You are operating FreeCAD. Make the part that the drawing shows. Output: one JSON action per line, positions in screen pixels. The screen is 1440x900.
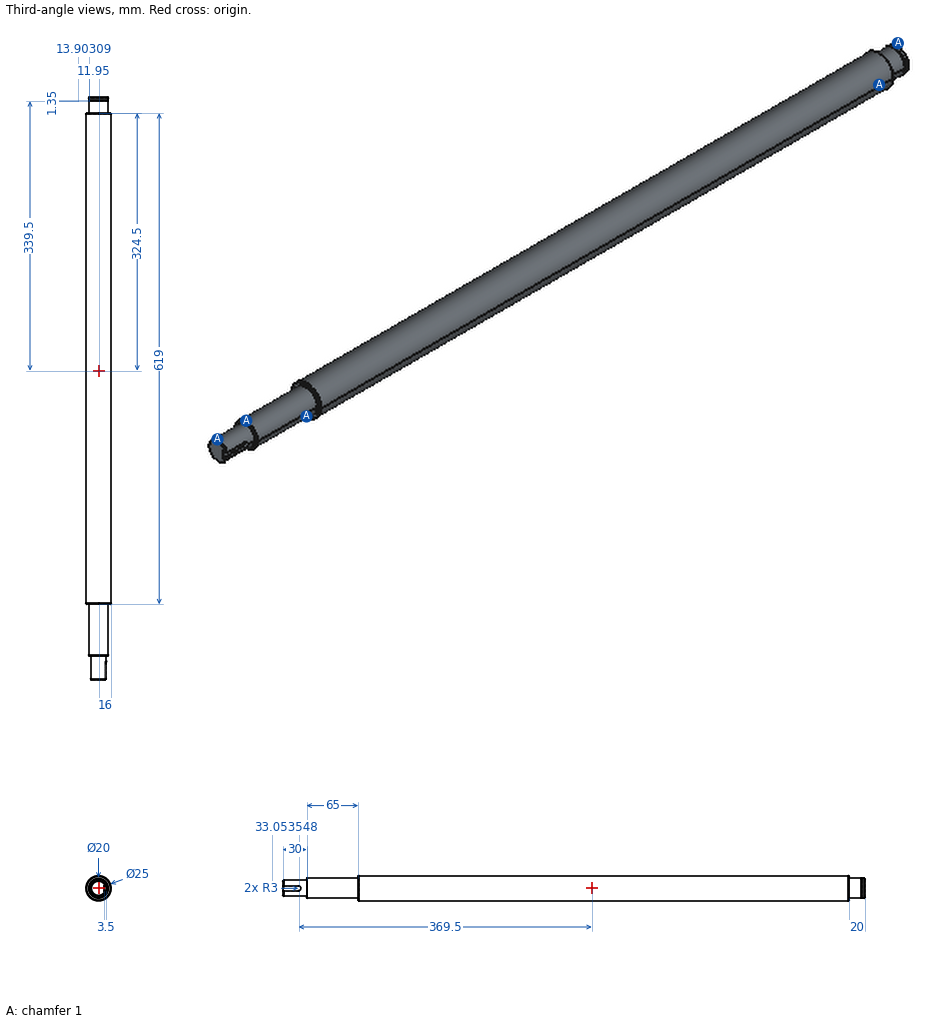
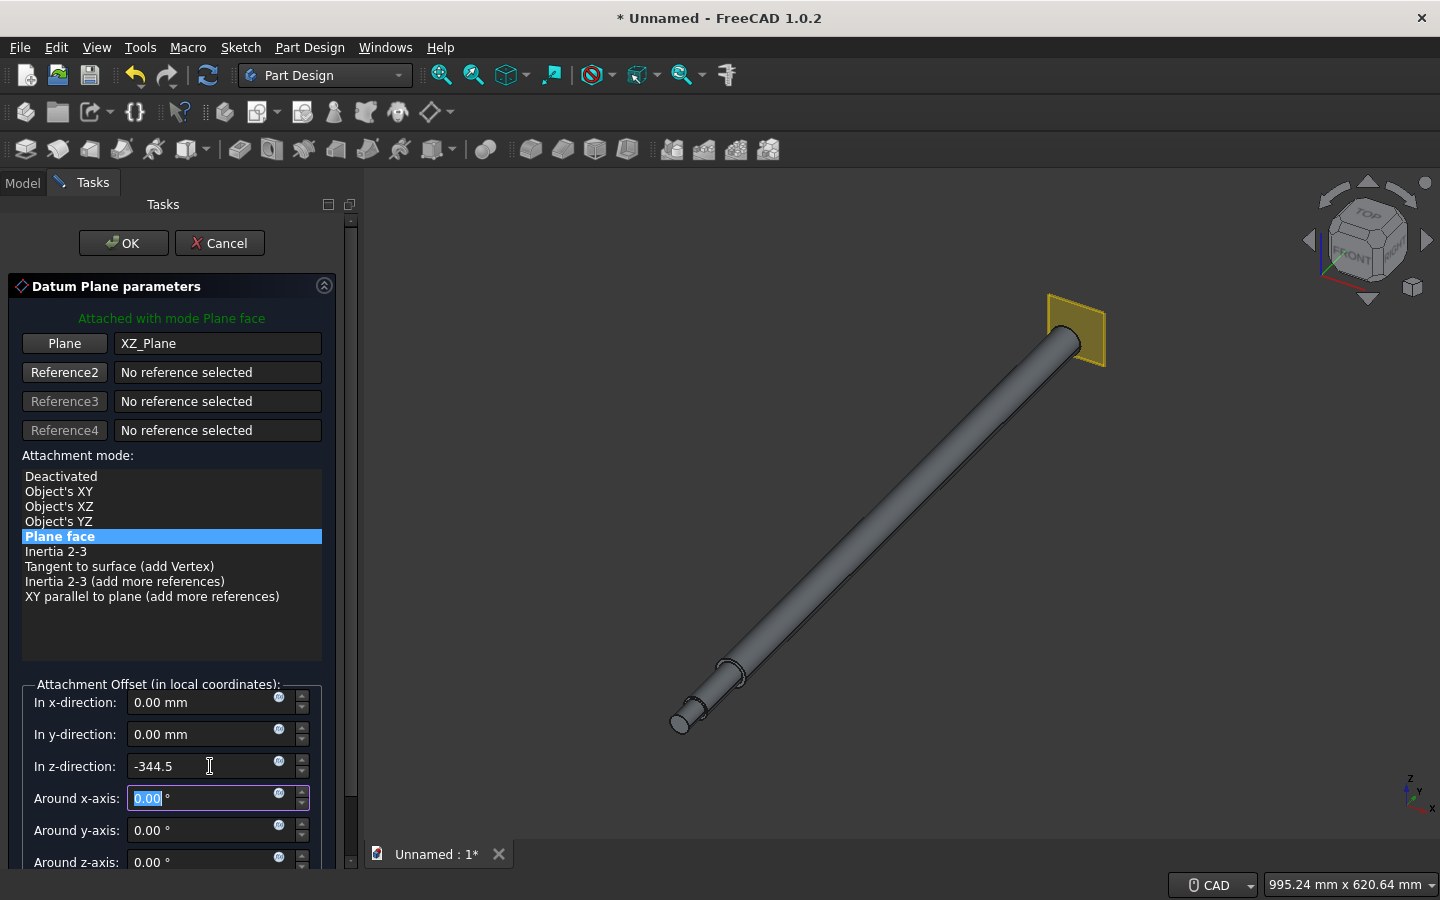
{"action": "left_click", "coordinate": [124, 243]}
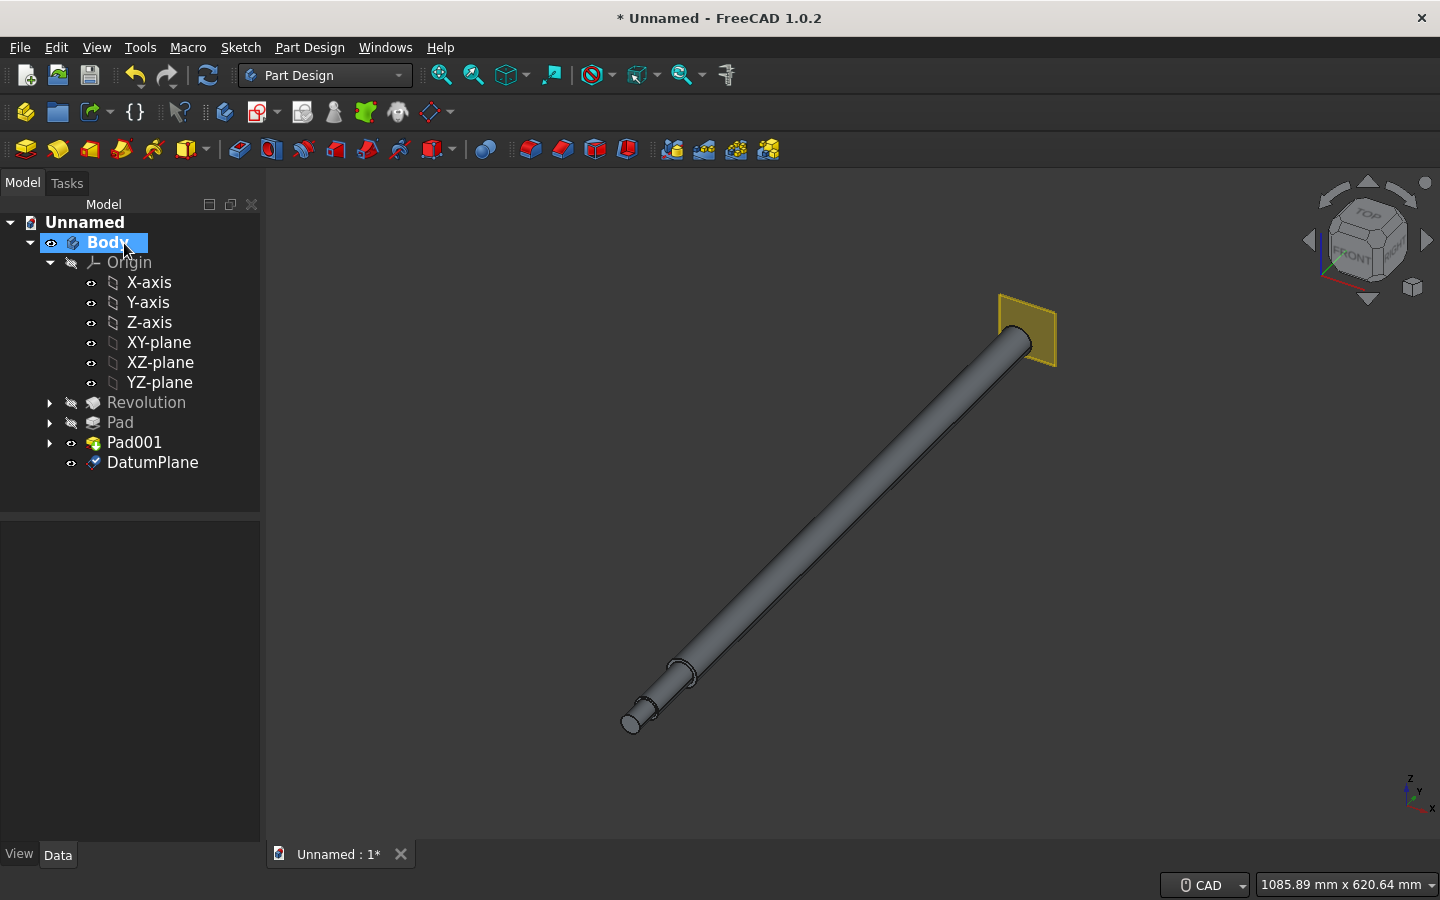
{"action": "left_click", "coordinate": [116, 463]}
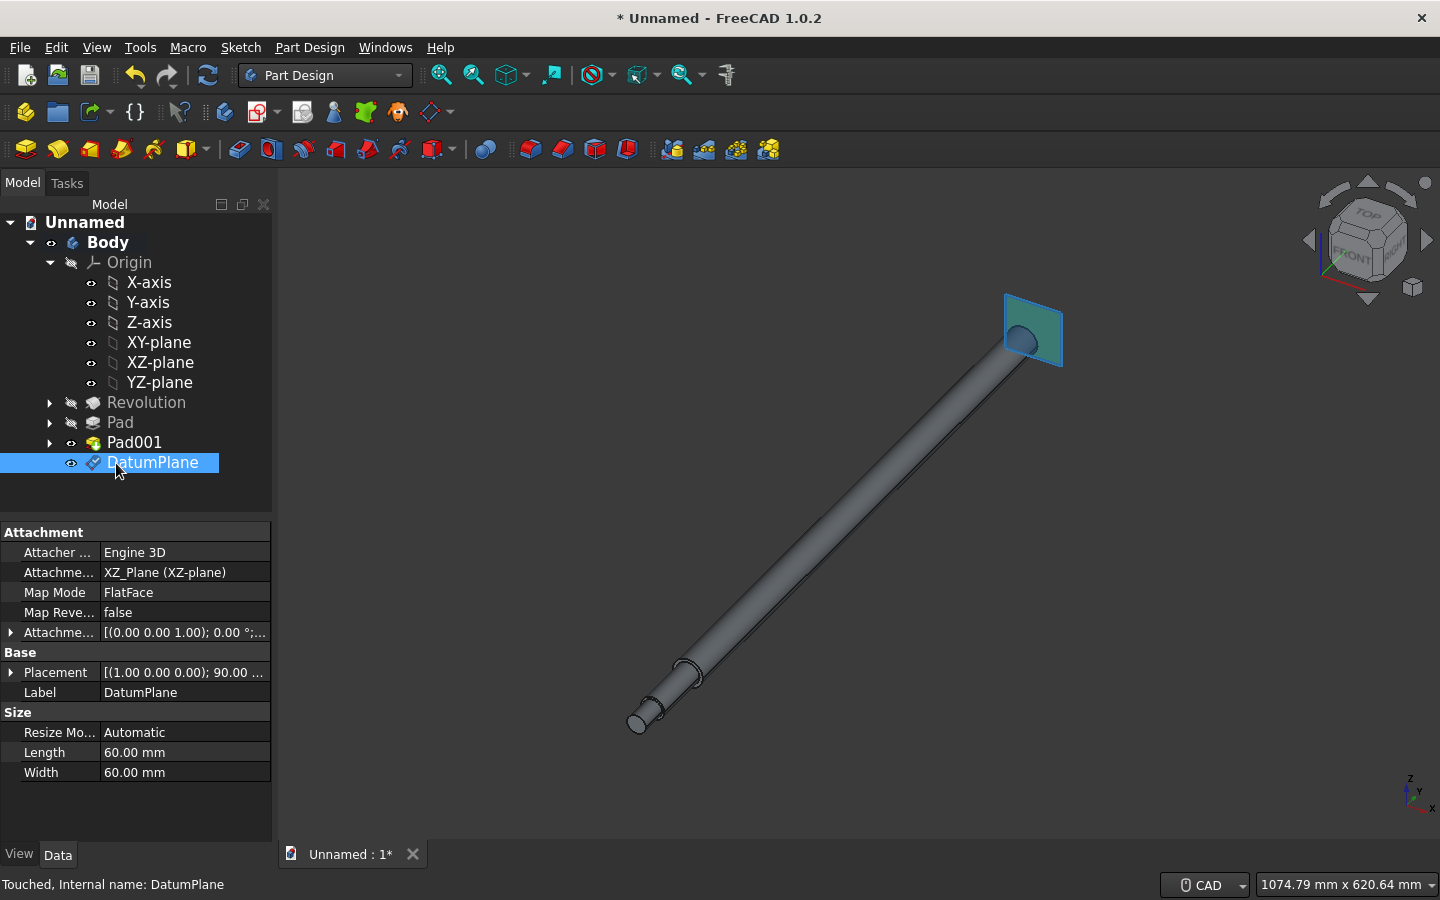
{"action": "left_click", "coordinate": [258, 112]}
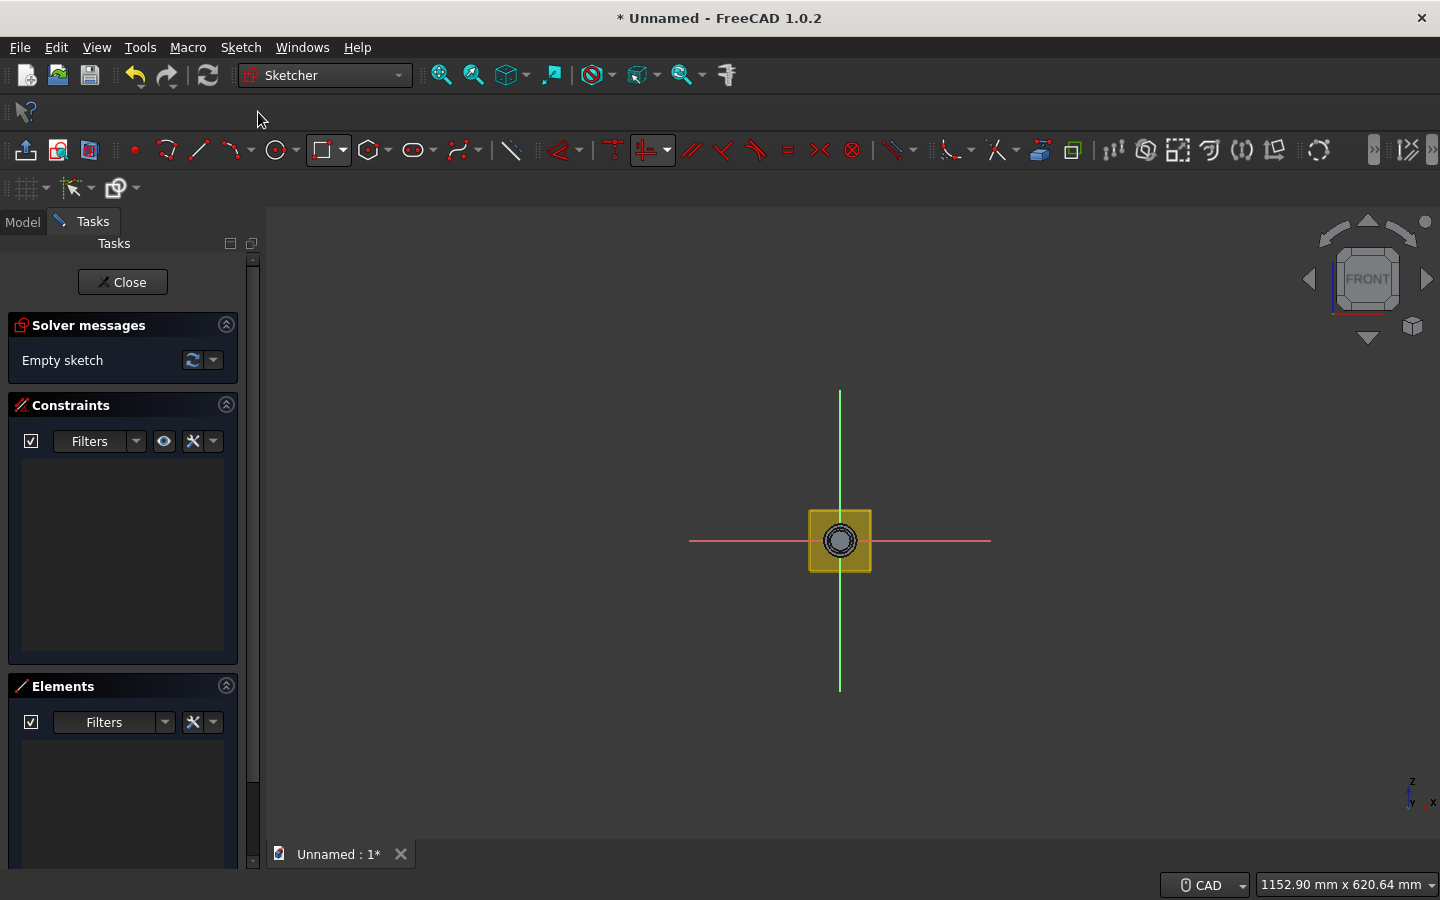
{"action": "left_click", "coordinate": [90, 150]}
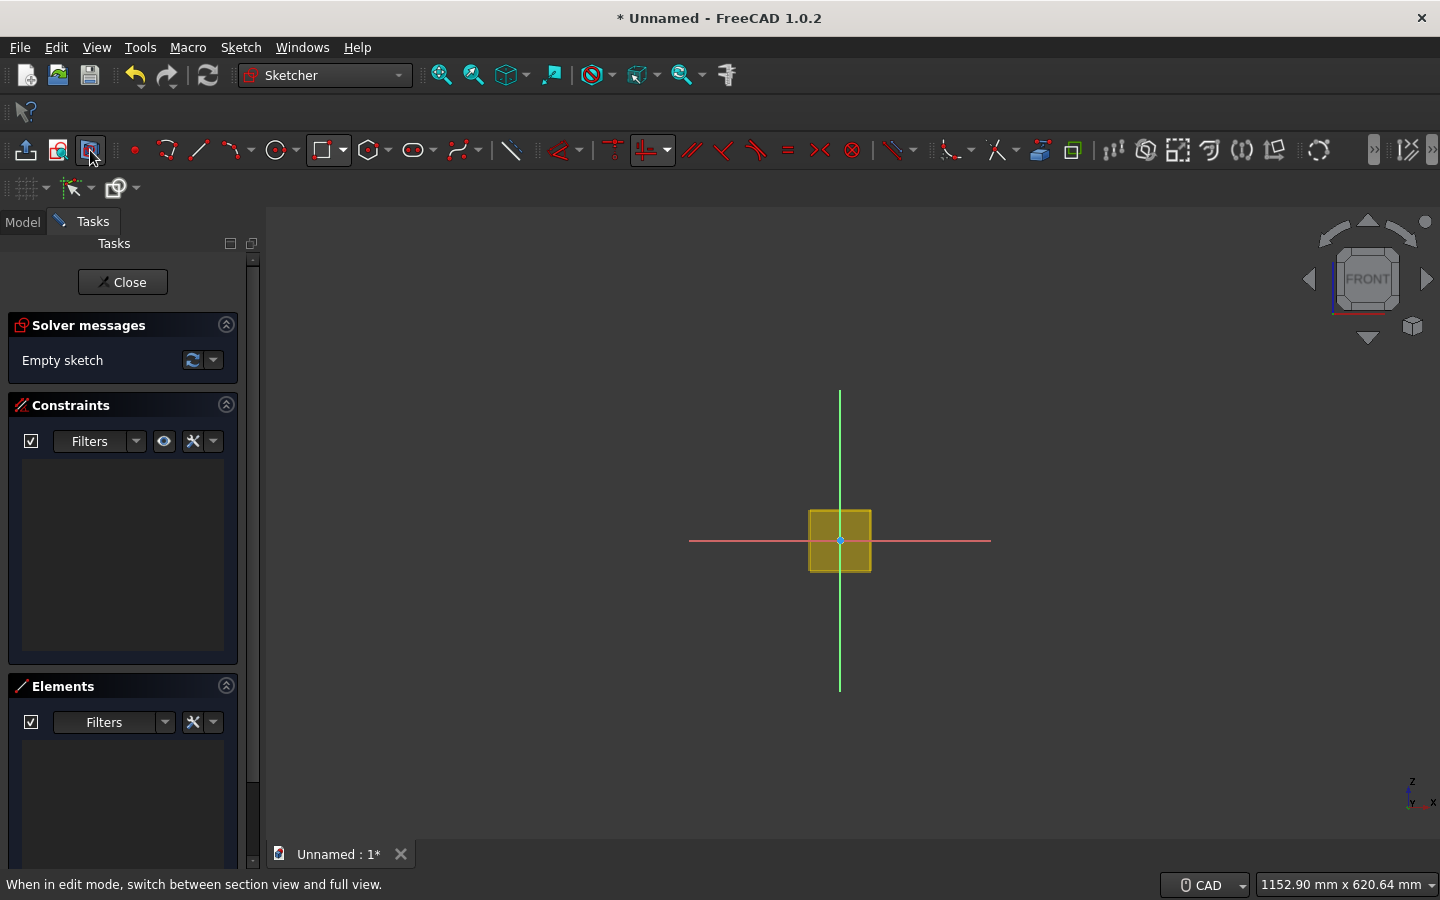
{"action": "scroll", "coordinate": [844, 542], "scroll_direction": "up", "scroll_amount": 14}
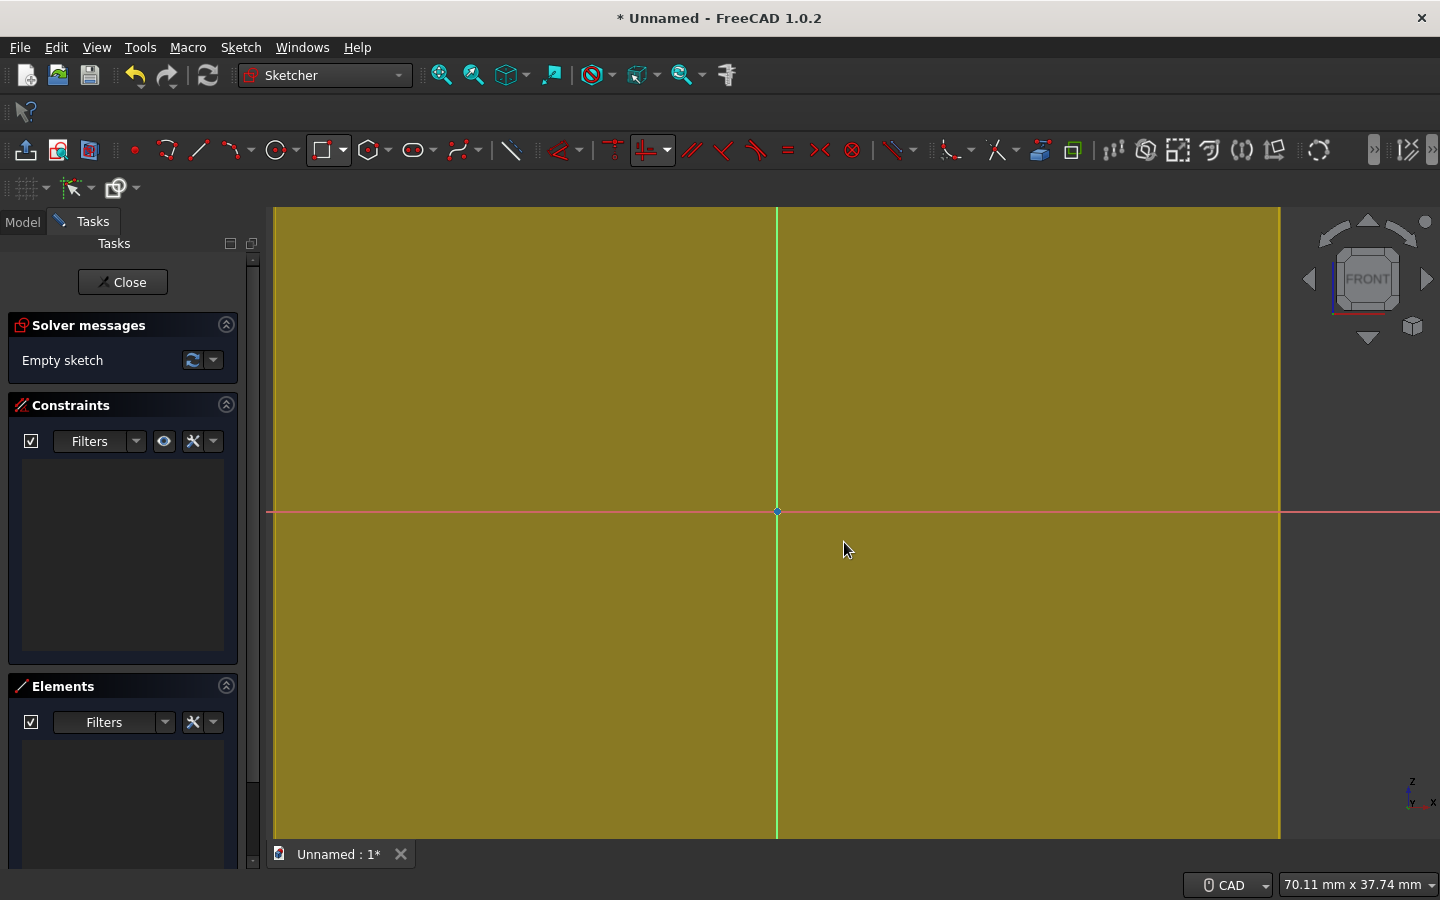
{"action": "left_click", "coordinate": [276, 150]}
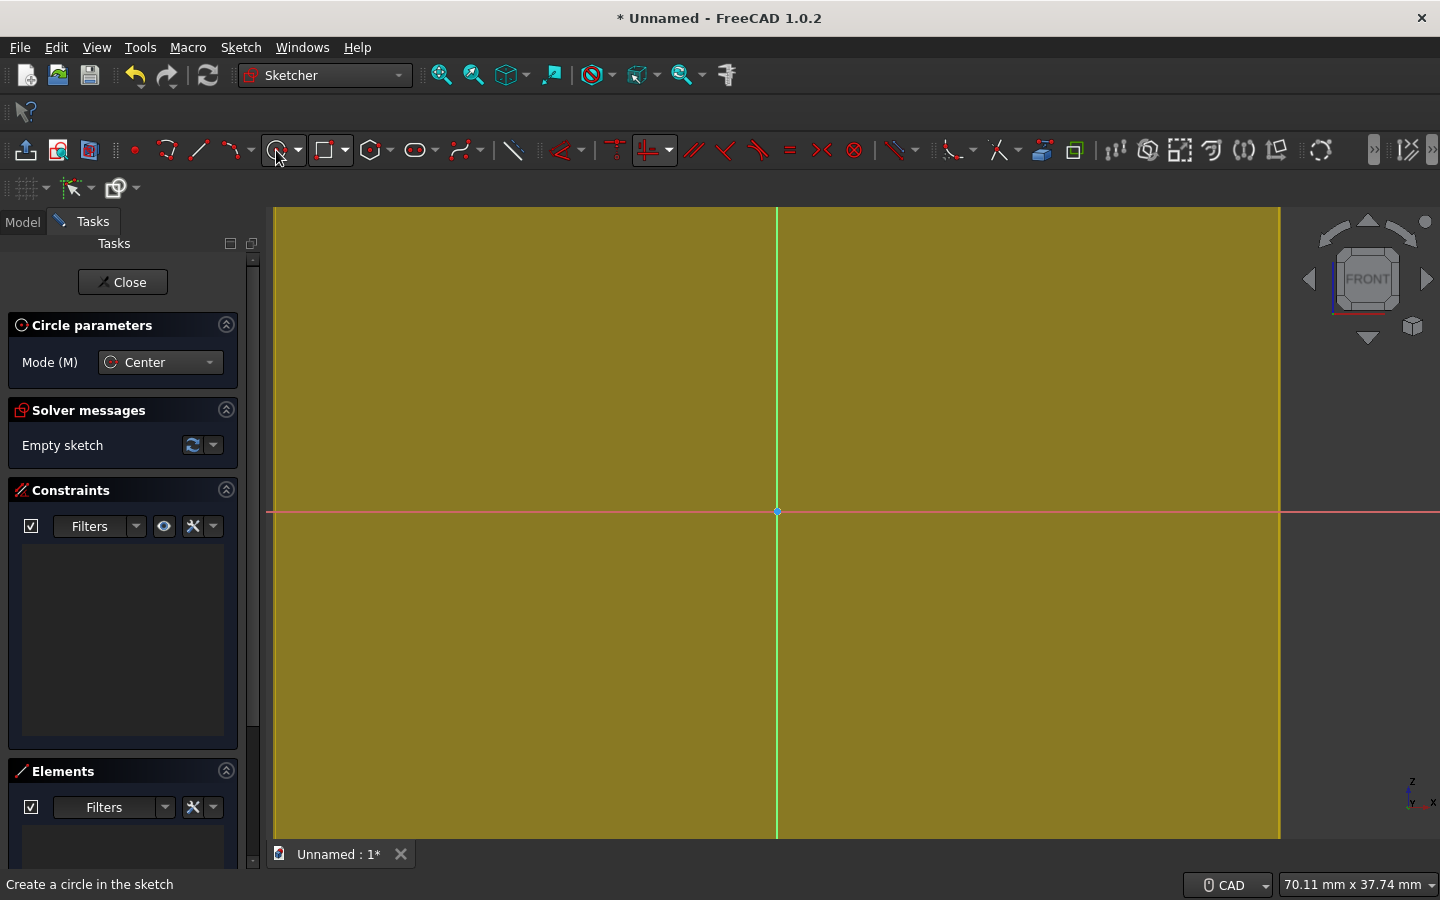
{"action": "left_click", "coordinate": [777, 512]}
{"action": "mouse_move", "coordinate": [925, 364]}